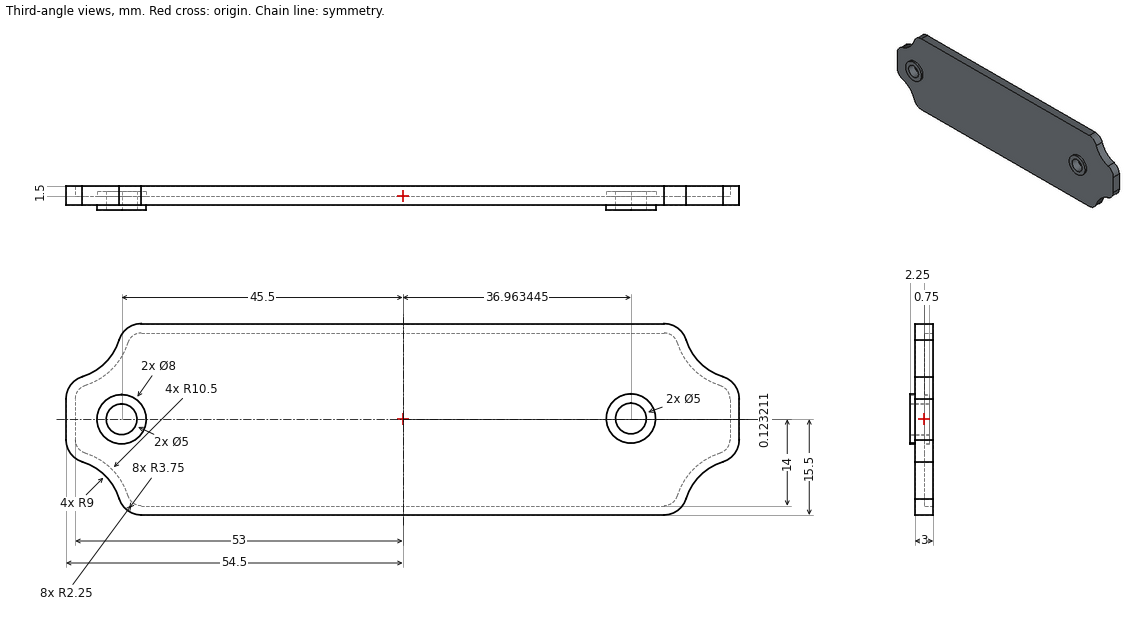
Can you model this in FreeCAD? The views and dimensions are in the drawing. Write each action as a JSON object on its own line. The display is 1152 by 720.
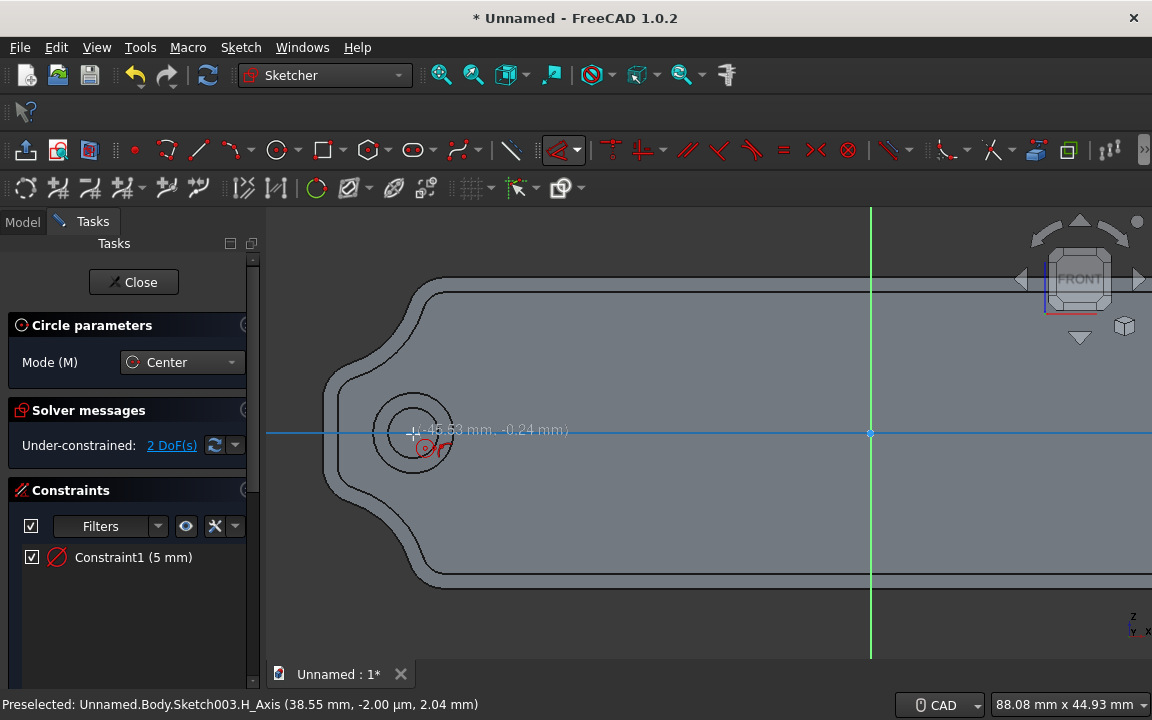
{"action": "left_click", "coordinate": [413, 433]}
{"action": "mouse_move", "coordinate": [431, 415]}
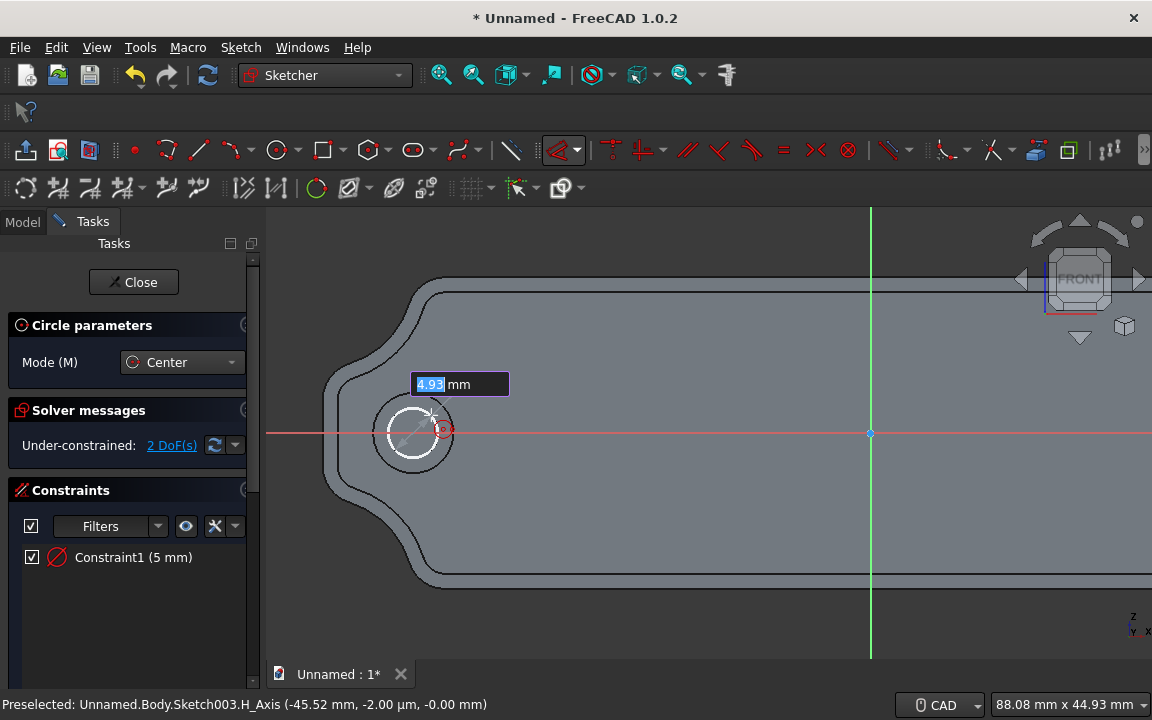
{"action": "type", "text": "5"}
{"action": "key", "text": "Return"}
{"action": "key", "text": "Escape"}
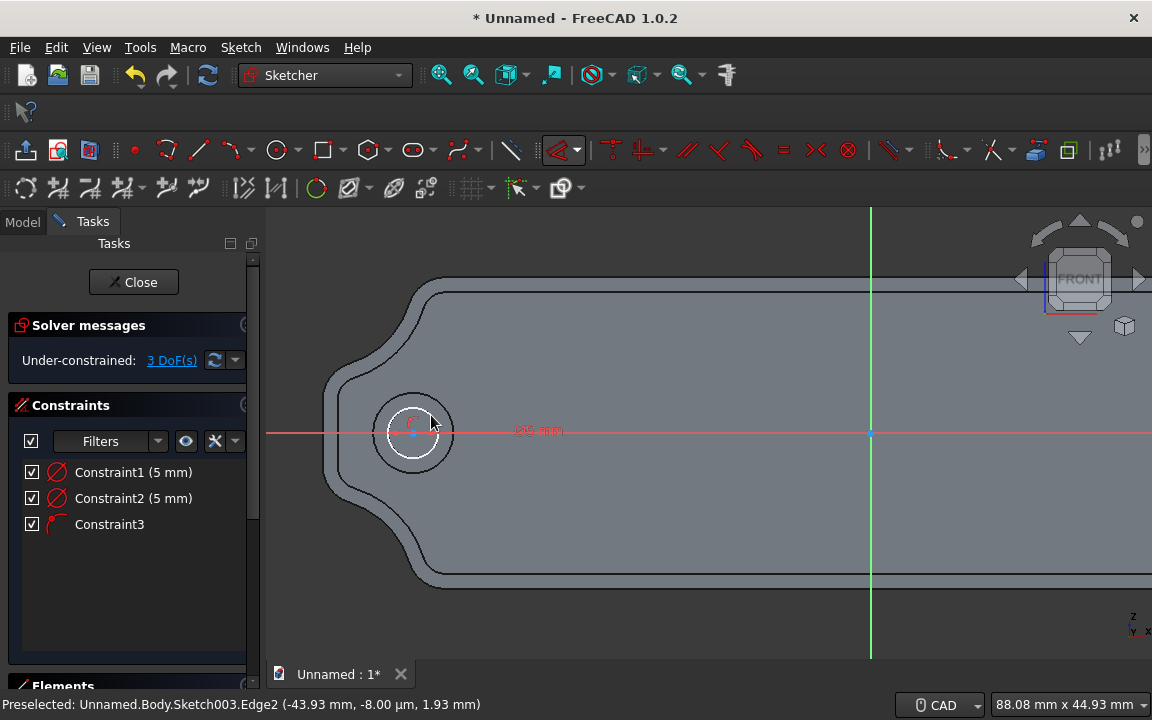
{"action": "left_click", "coordinate": [413, 433]}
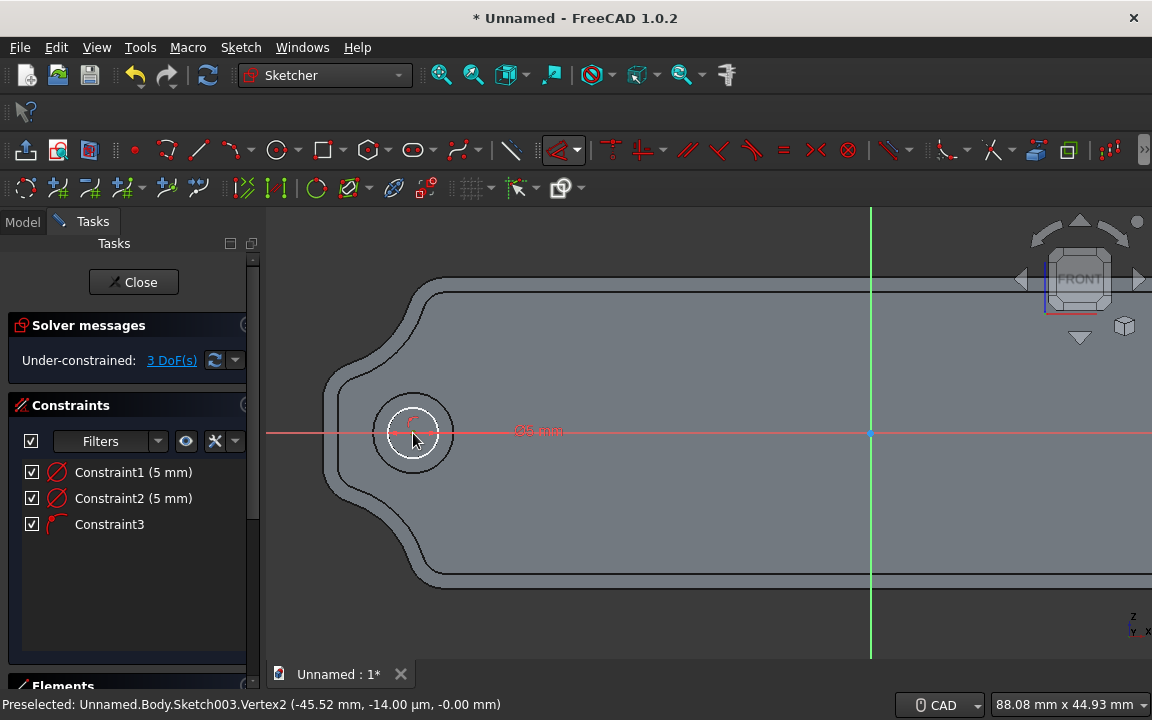
{"action": "left_click", "coordinate": [580, 150]}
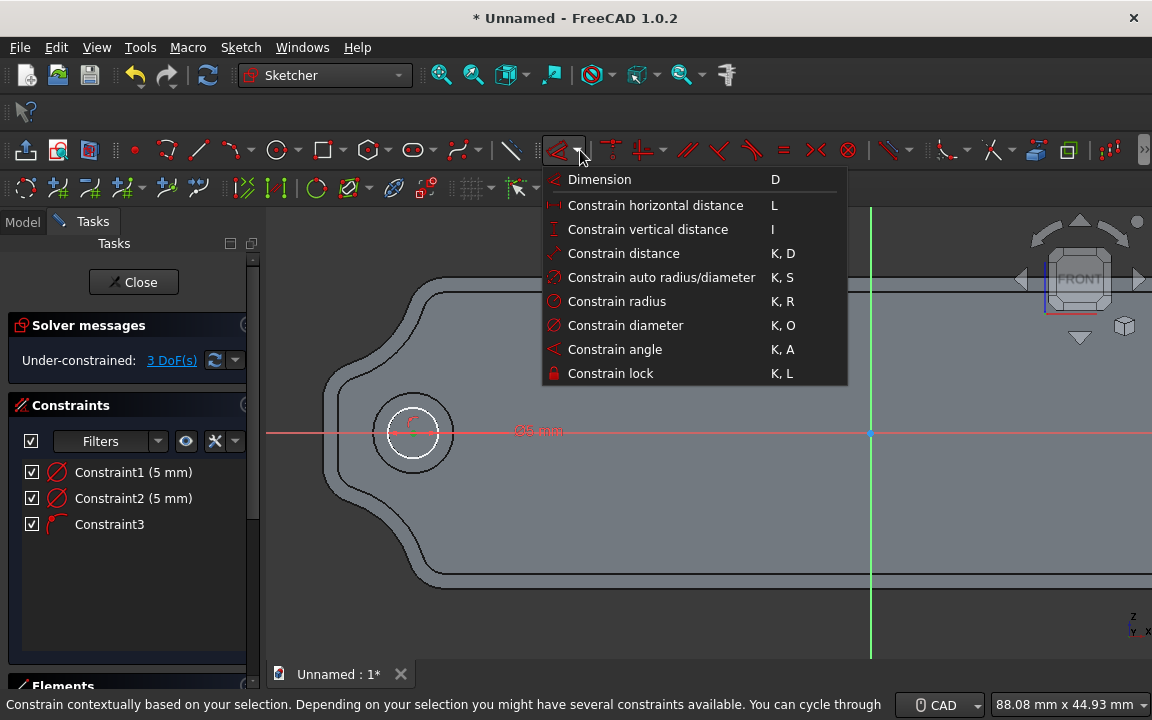
{"action": "left_click", "coordinate": [695, 205]}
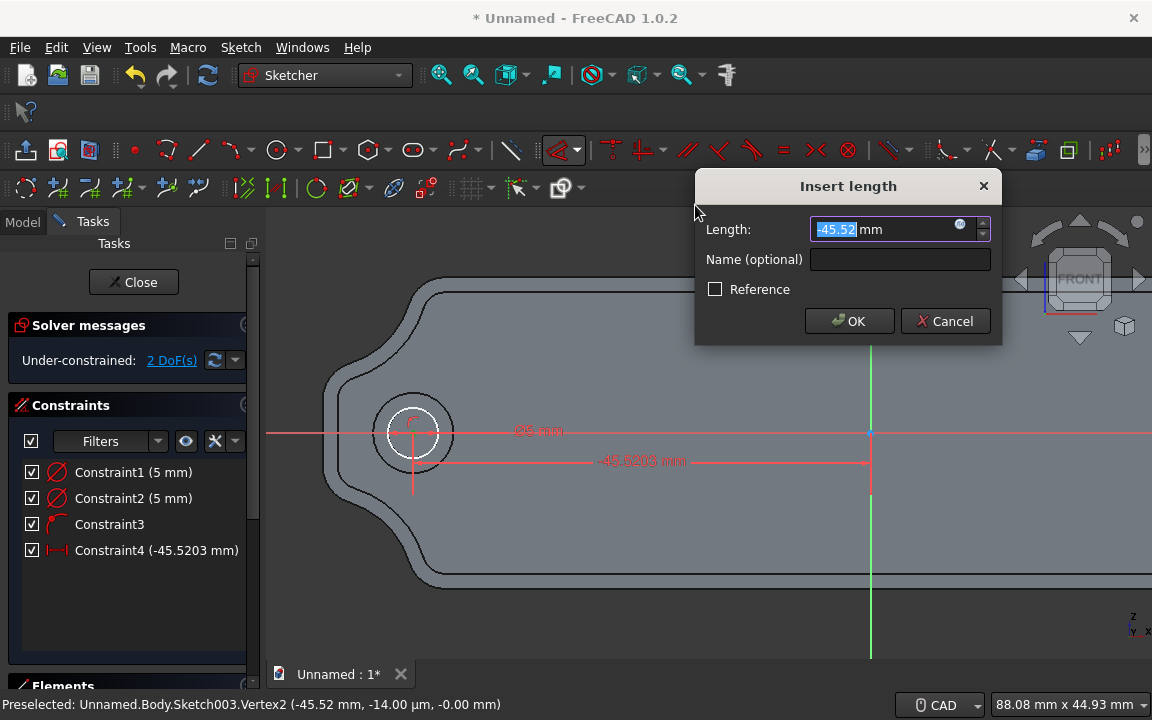
{"action": "type", "text": "-45.5"}
{"action": "key", "text": "Return"}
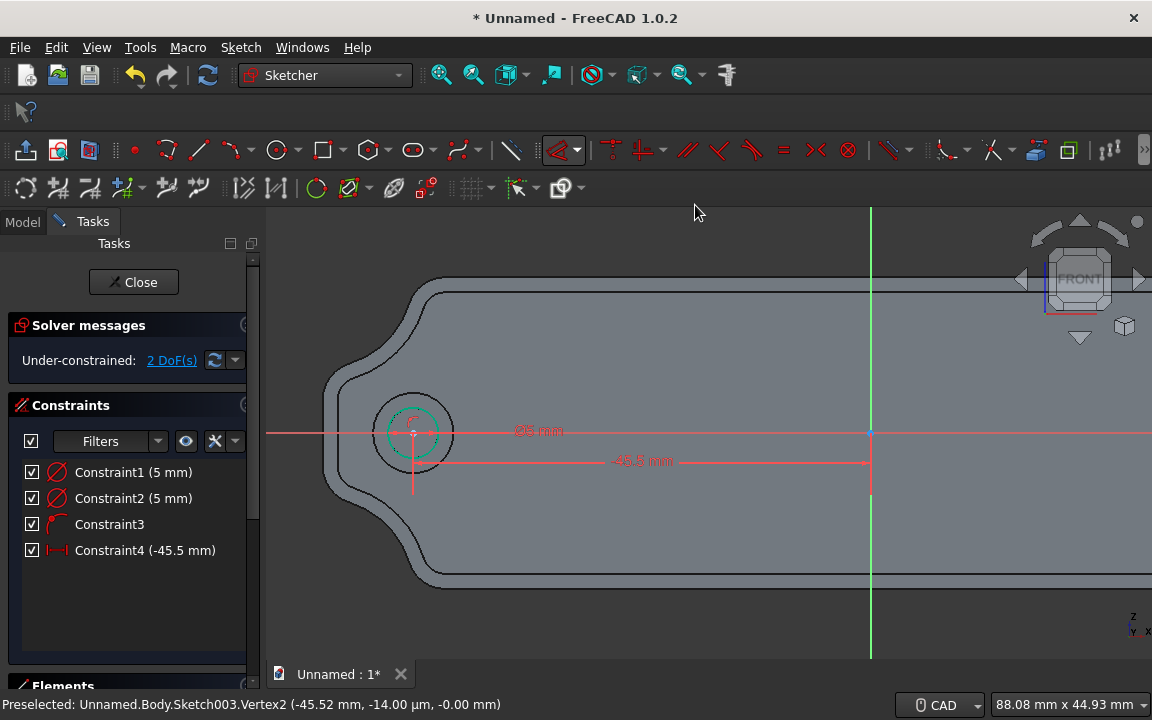
{"action": "scroll", "coordinate": [412, 434], "scroll_direction": "down", "scroll_amount": 3}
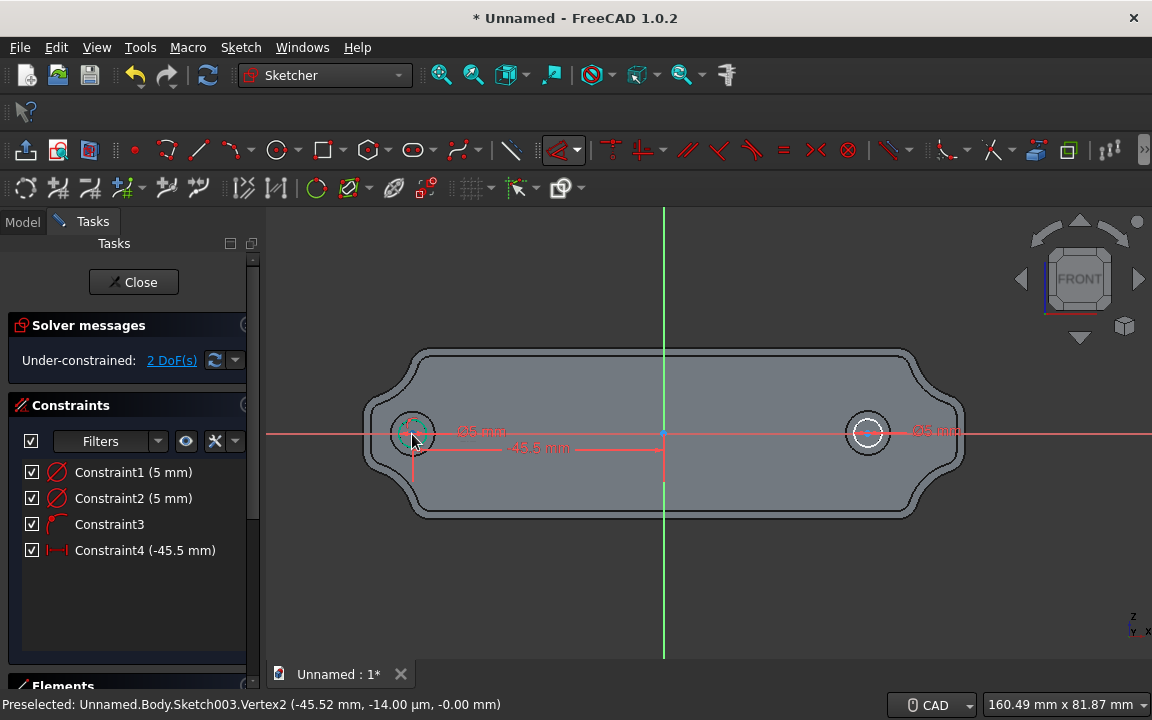
{"action": "scroll", "coordinate": [868, 433], "scroll_direction": "up", "scroll_amount": 21}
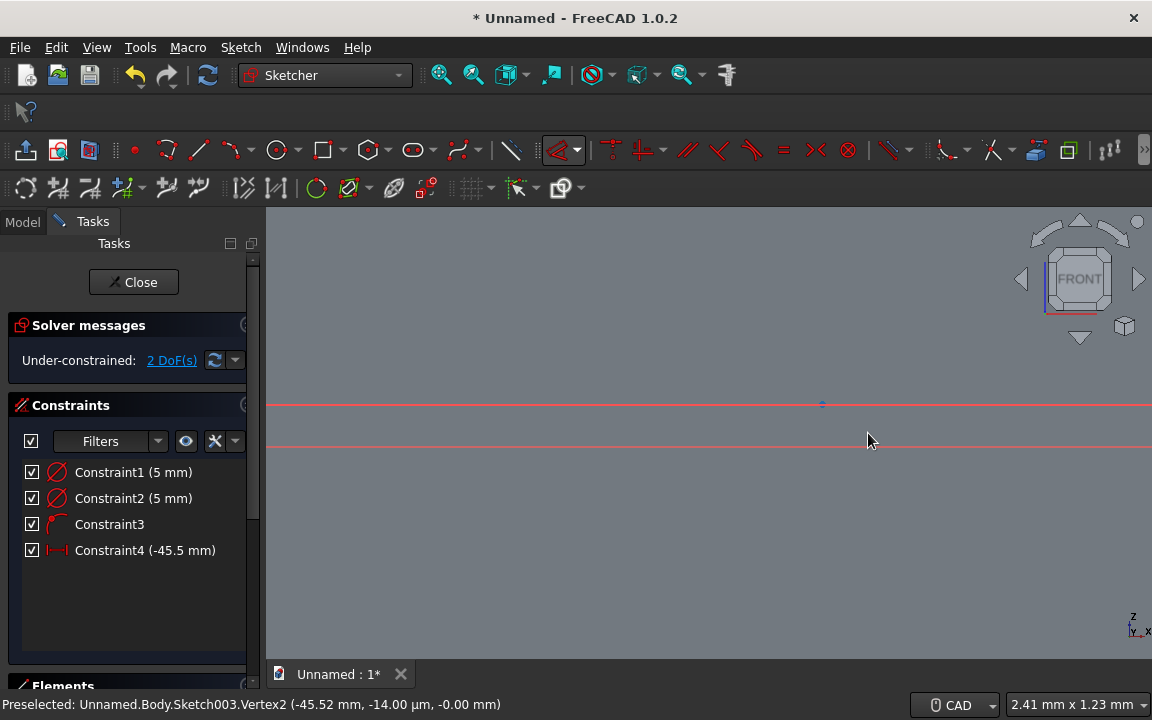
{"action": "left_click", "coordinate": [822, 405]}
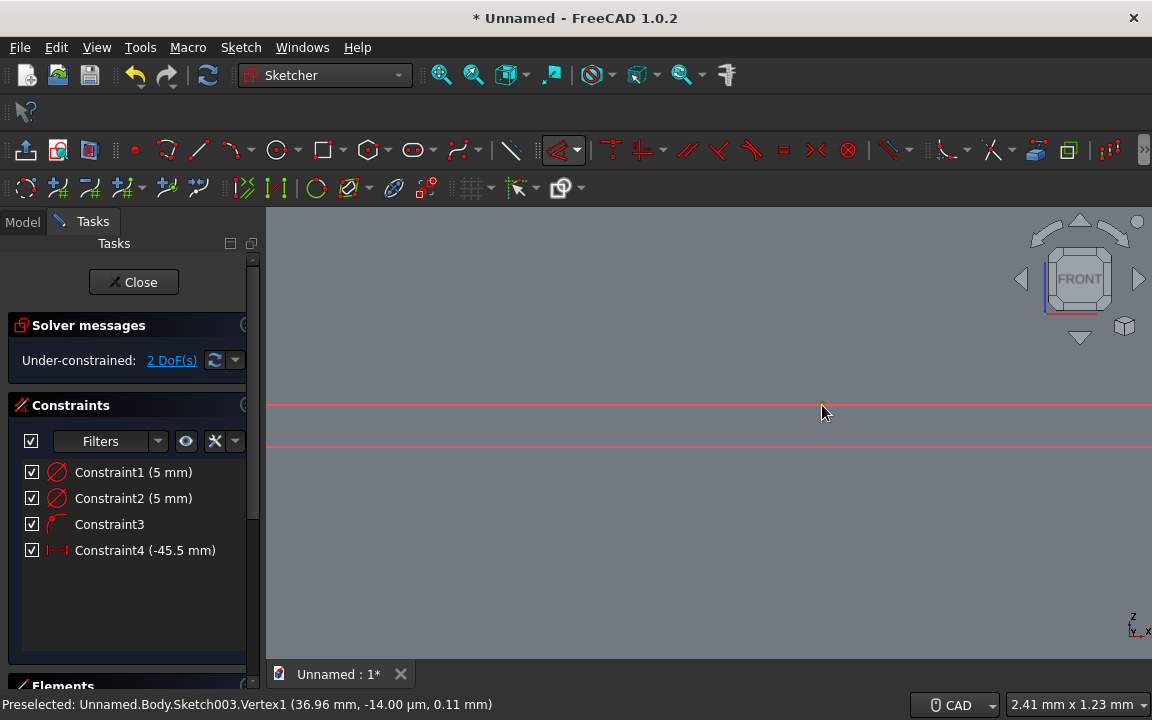
{"action": "key", "text": "i"}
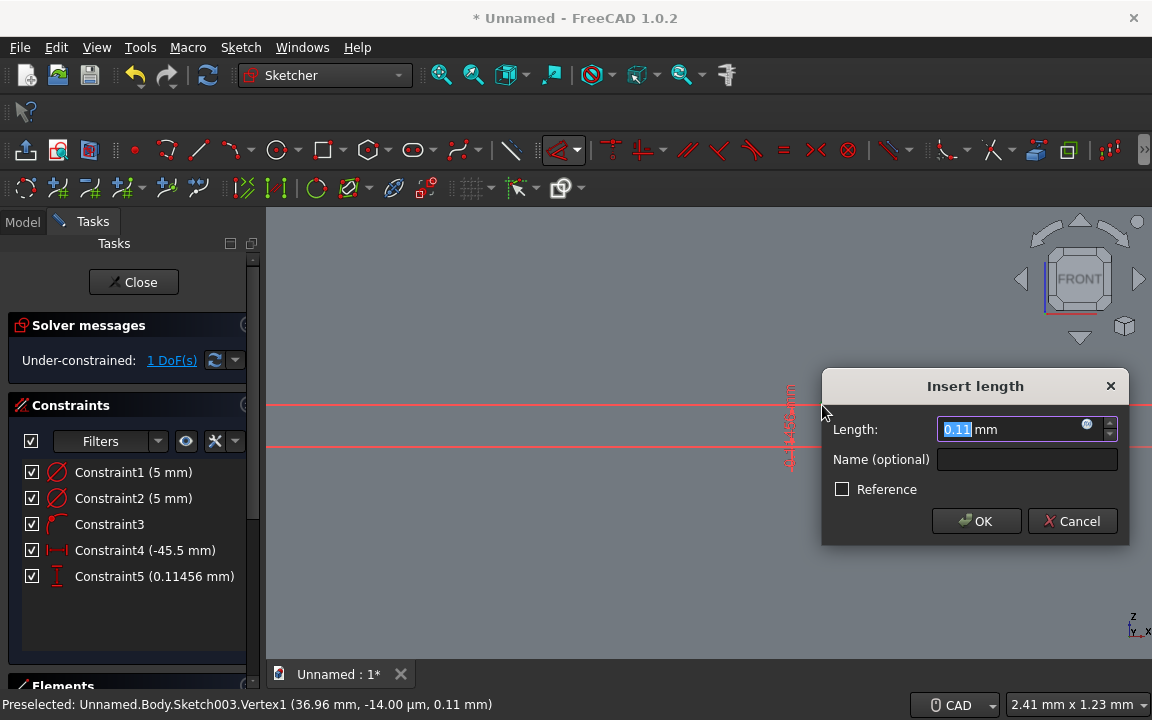
{"action": "type", "text": "0.123211"}
{"action": "key", "text": "Return"}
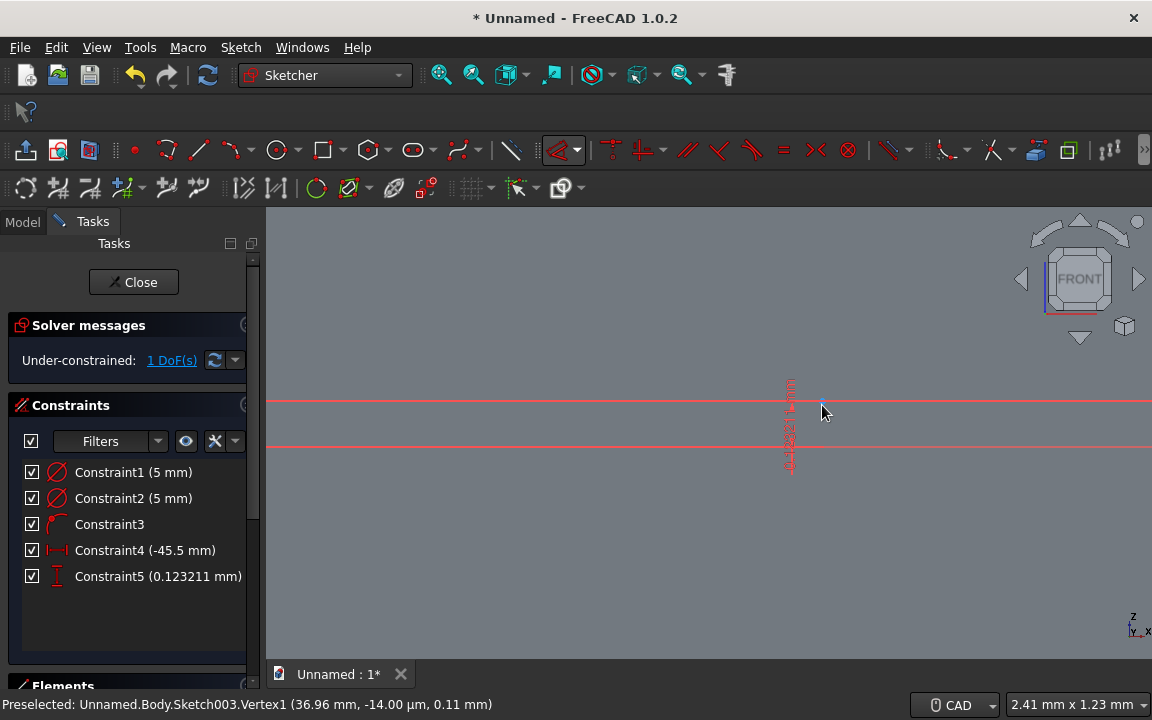
{"action": "scroll", "coordinate": [640, 433], "scroll_direction": "down", "scroll_amount": 15}